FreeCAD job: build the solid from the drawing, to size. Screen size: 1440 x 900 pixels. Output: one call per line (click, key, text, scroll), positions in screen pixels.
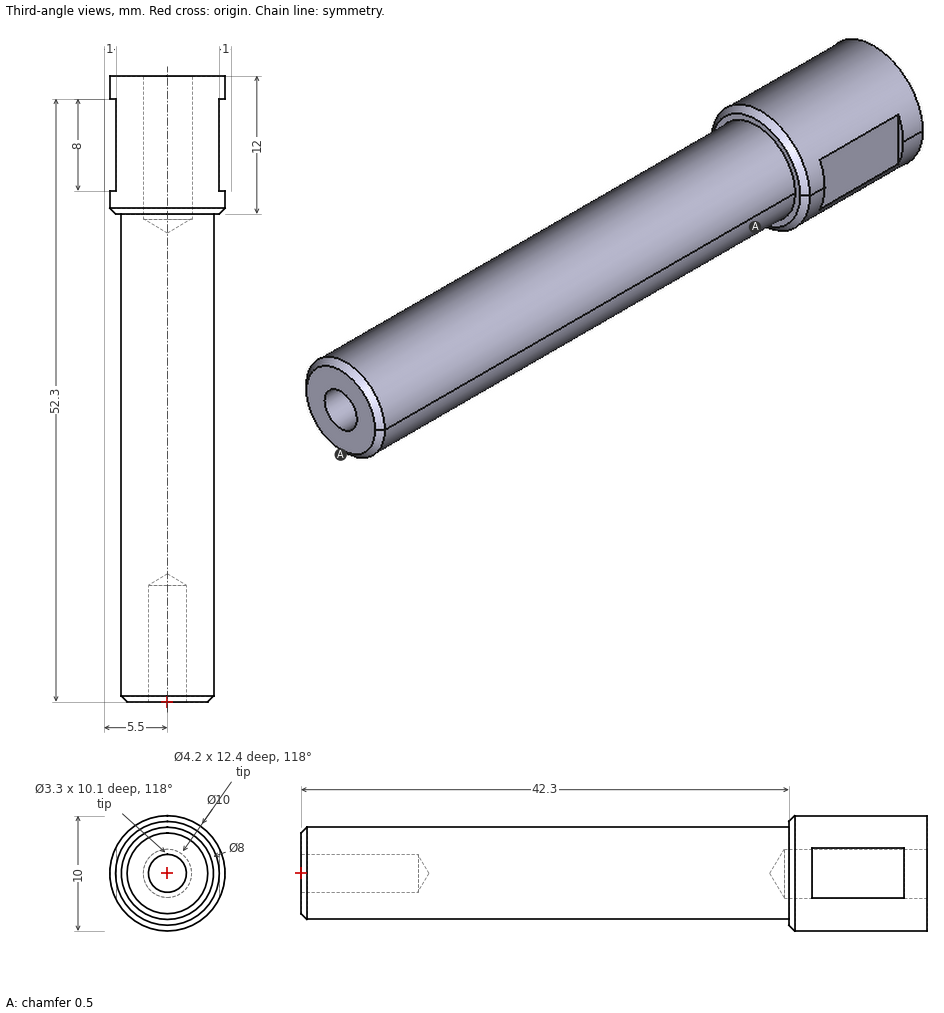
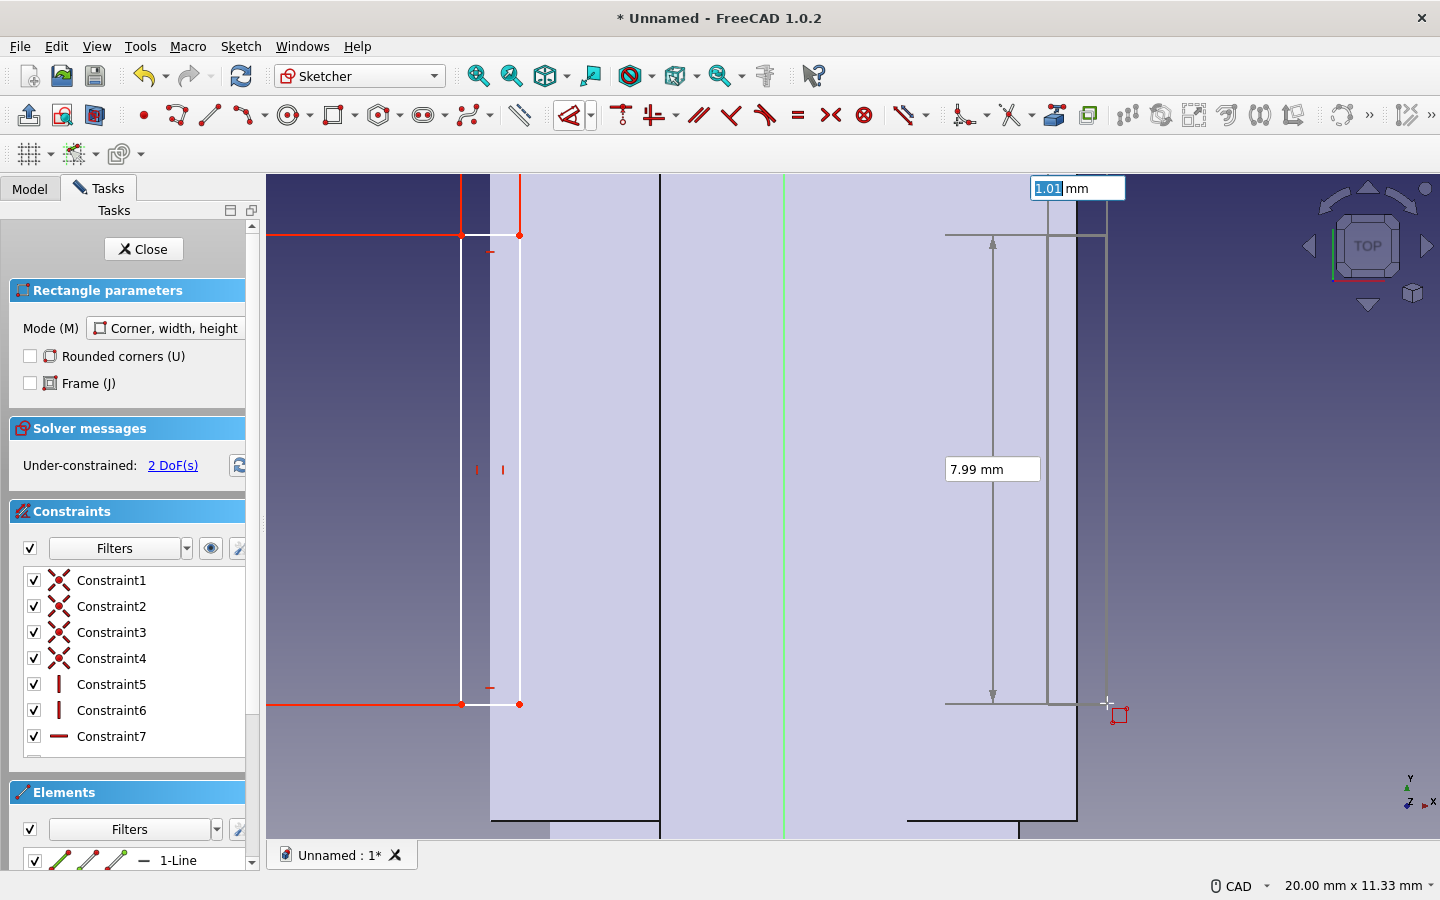
text(1)
key(Tab)
text(8)
key(Return)
key(Escape)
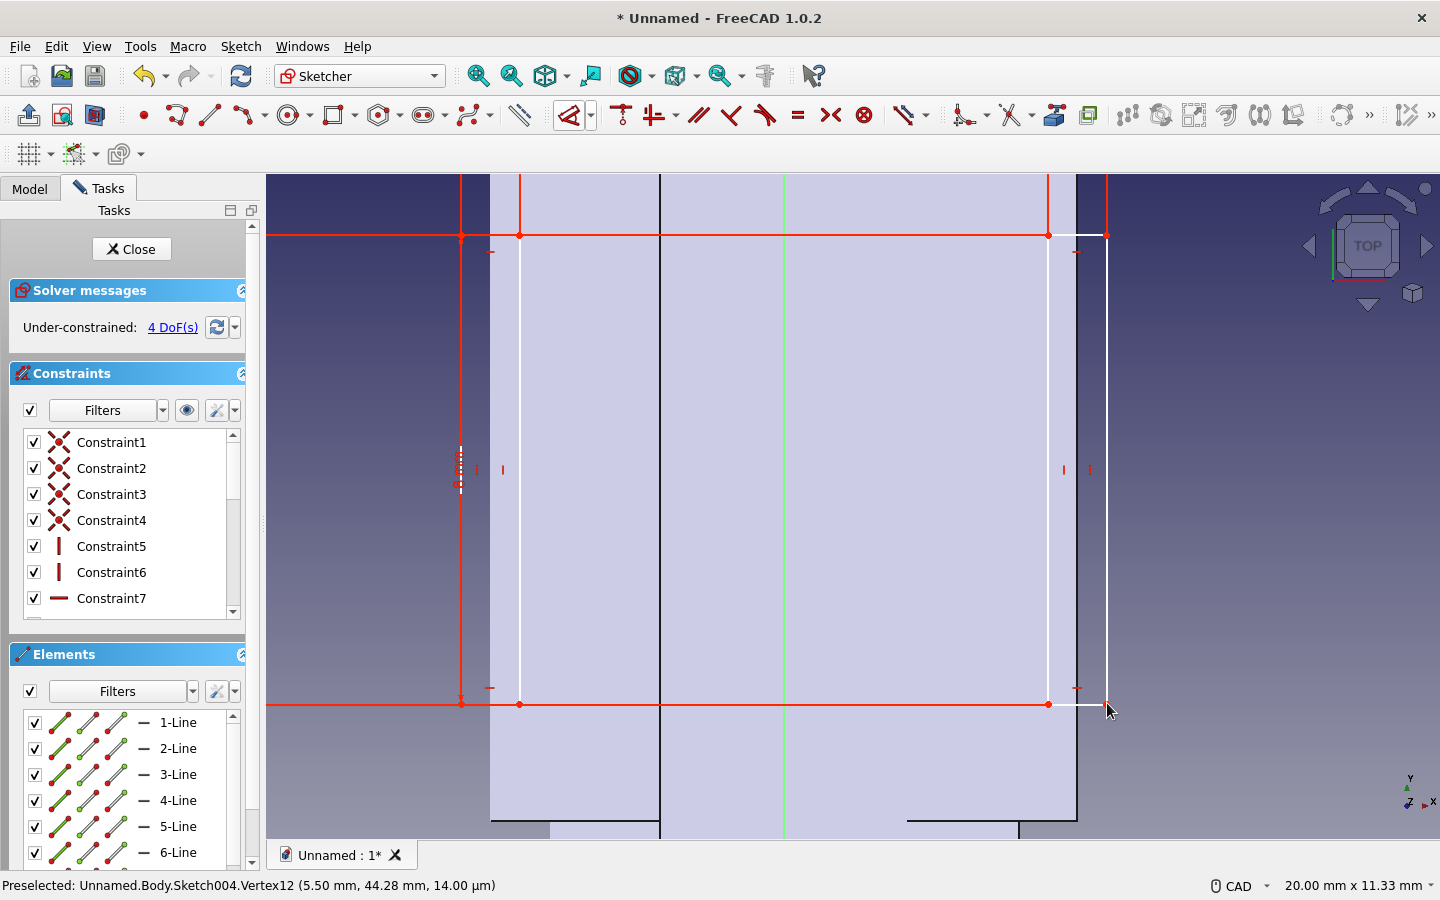
click(520, 235)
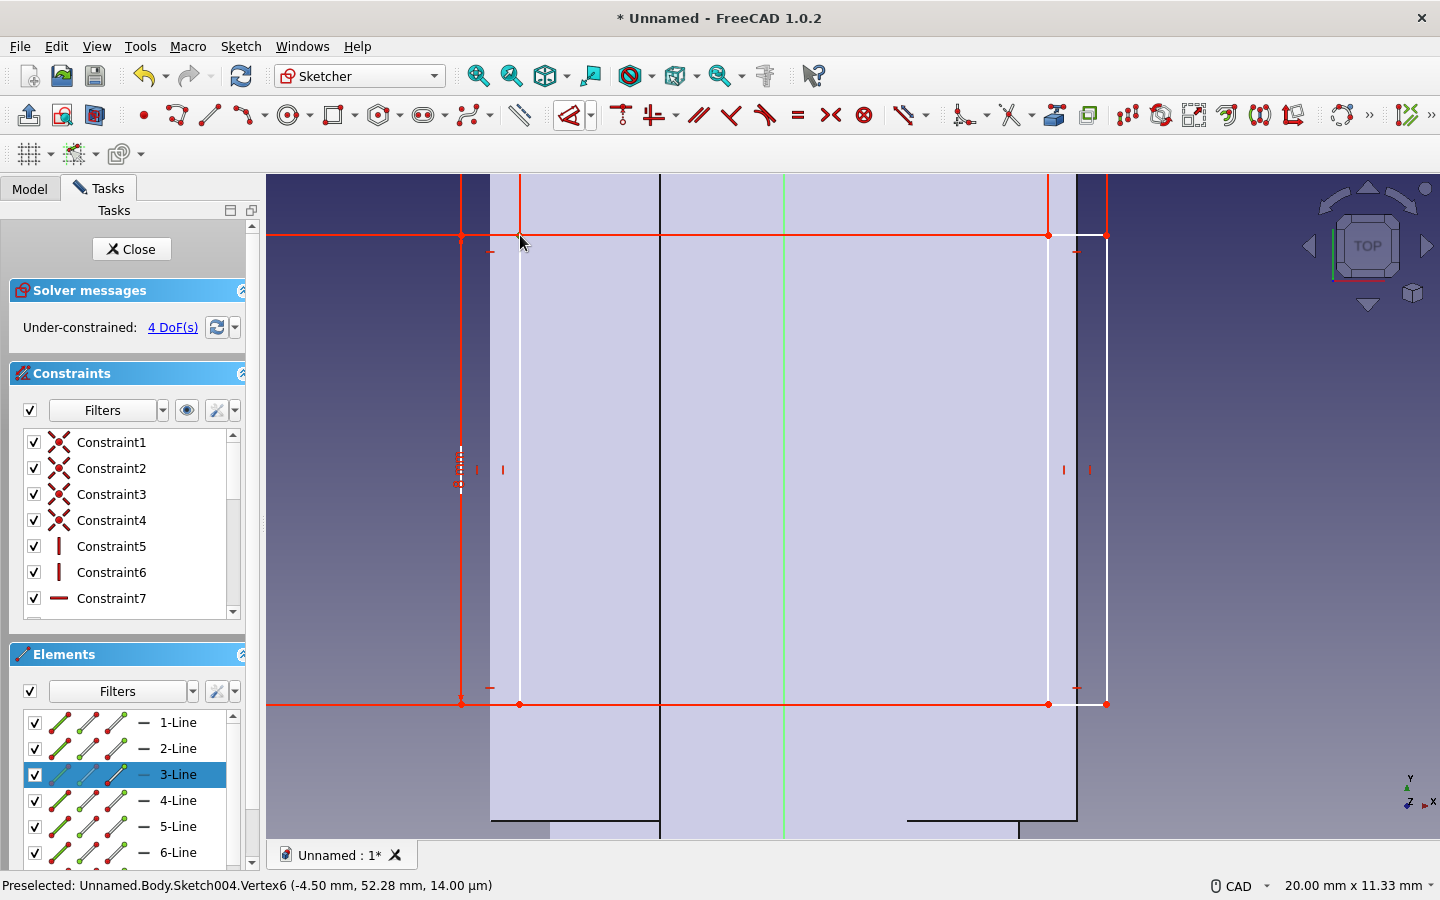
click(1048, 235)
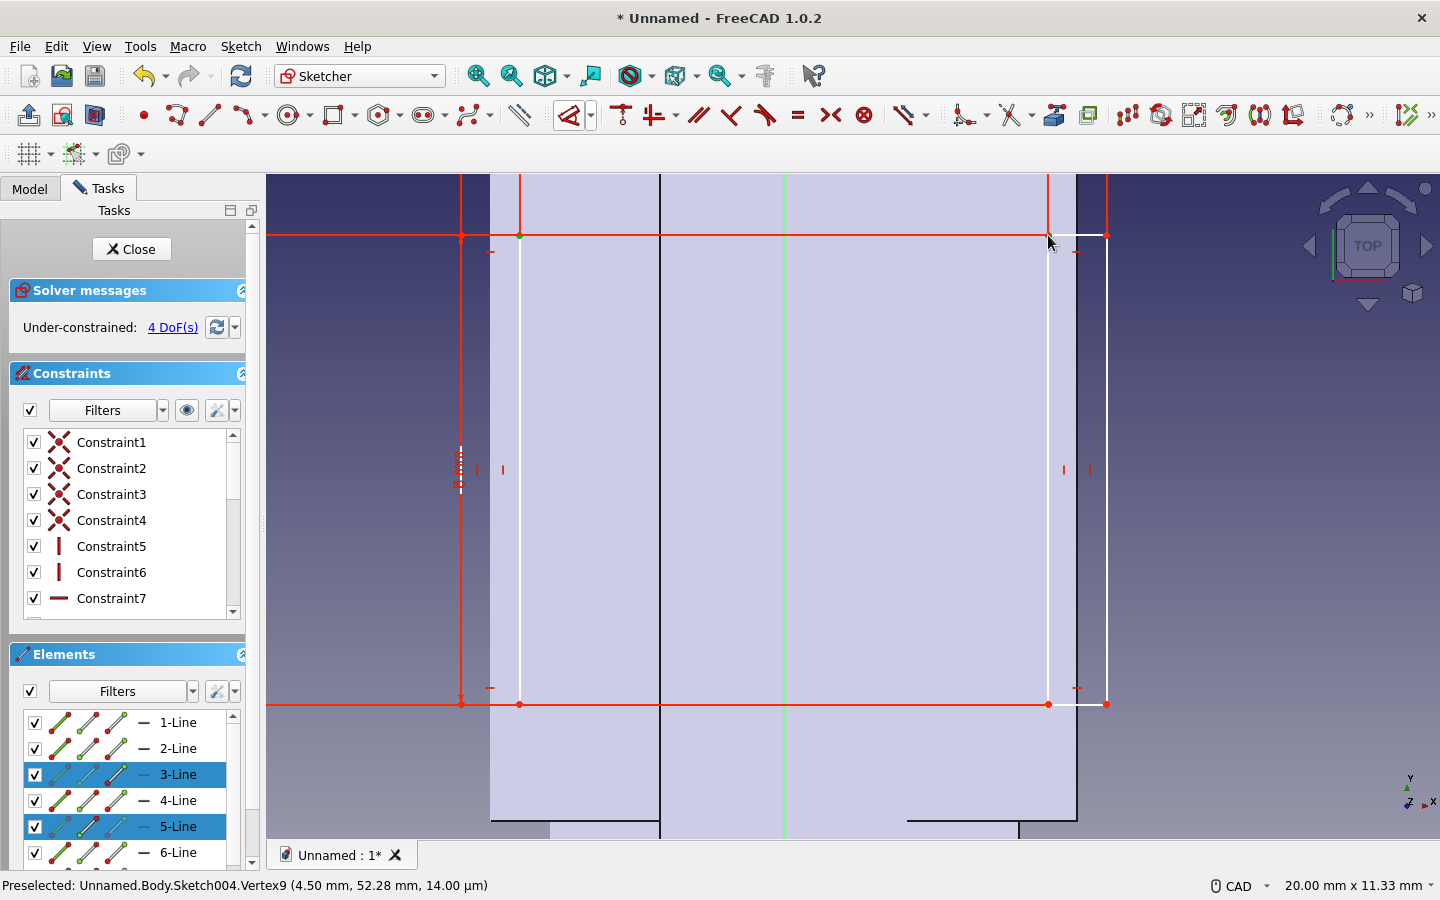
click(784, 767)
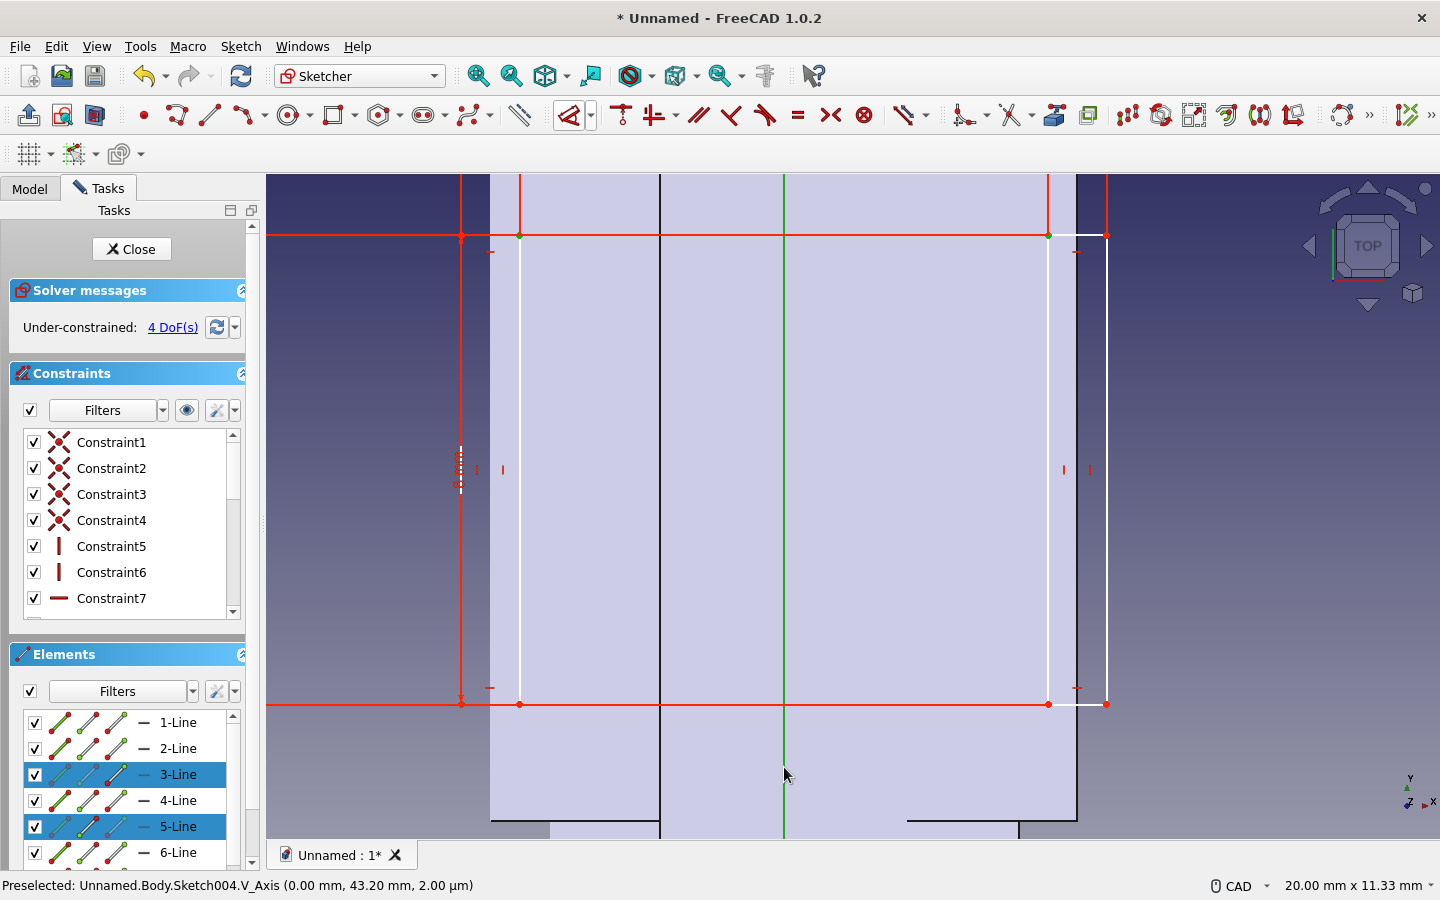
key(s)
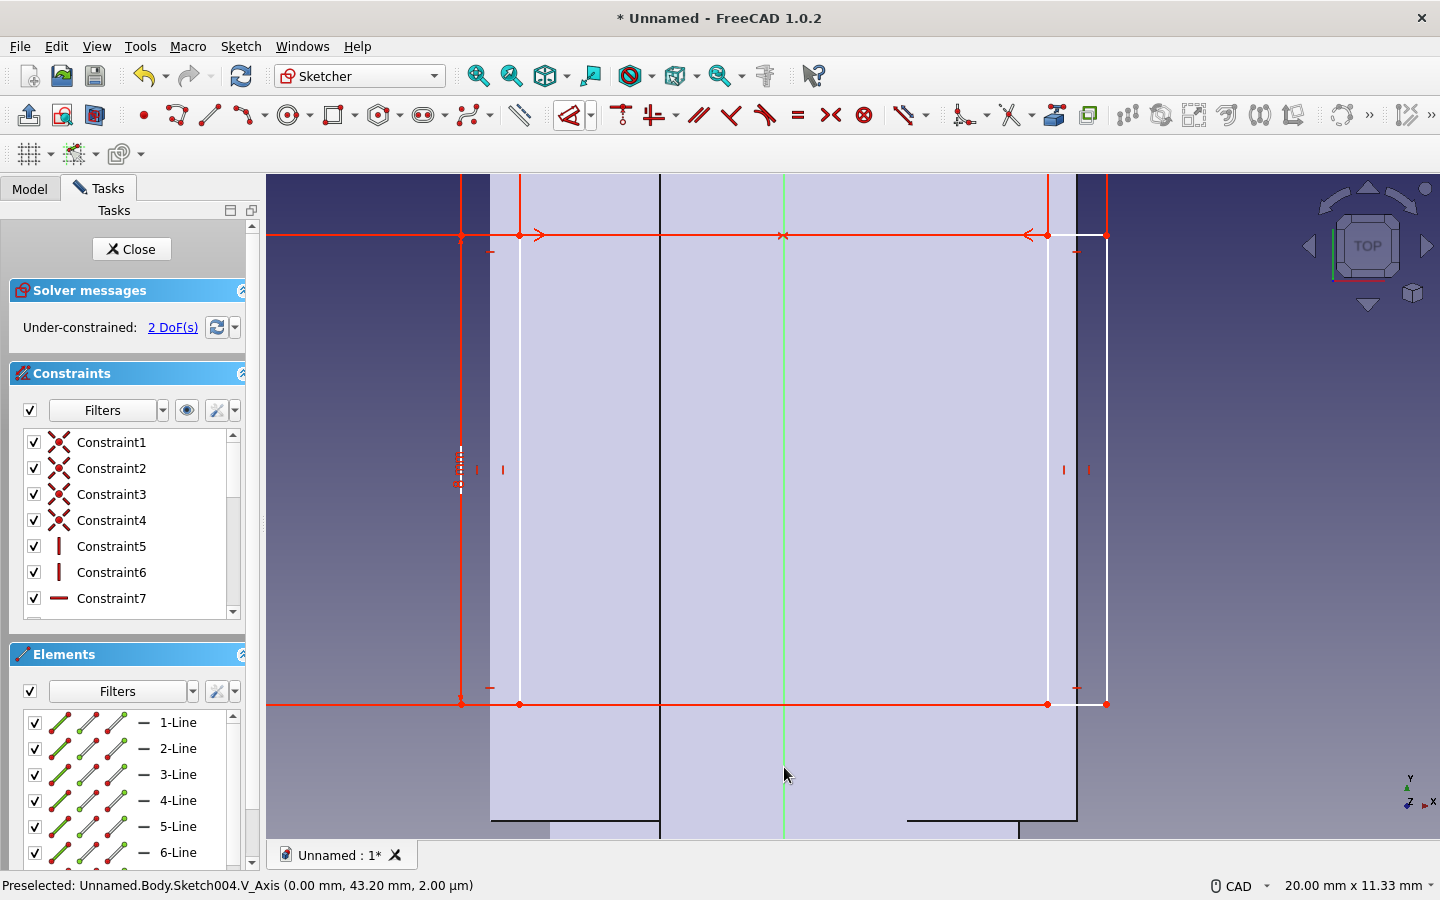
key(d)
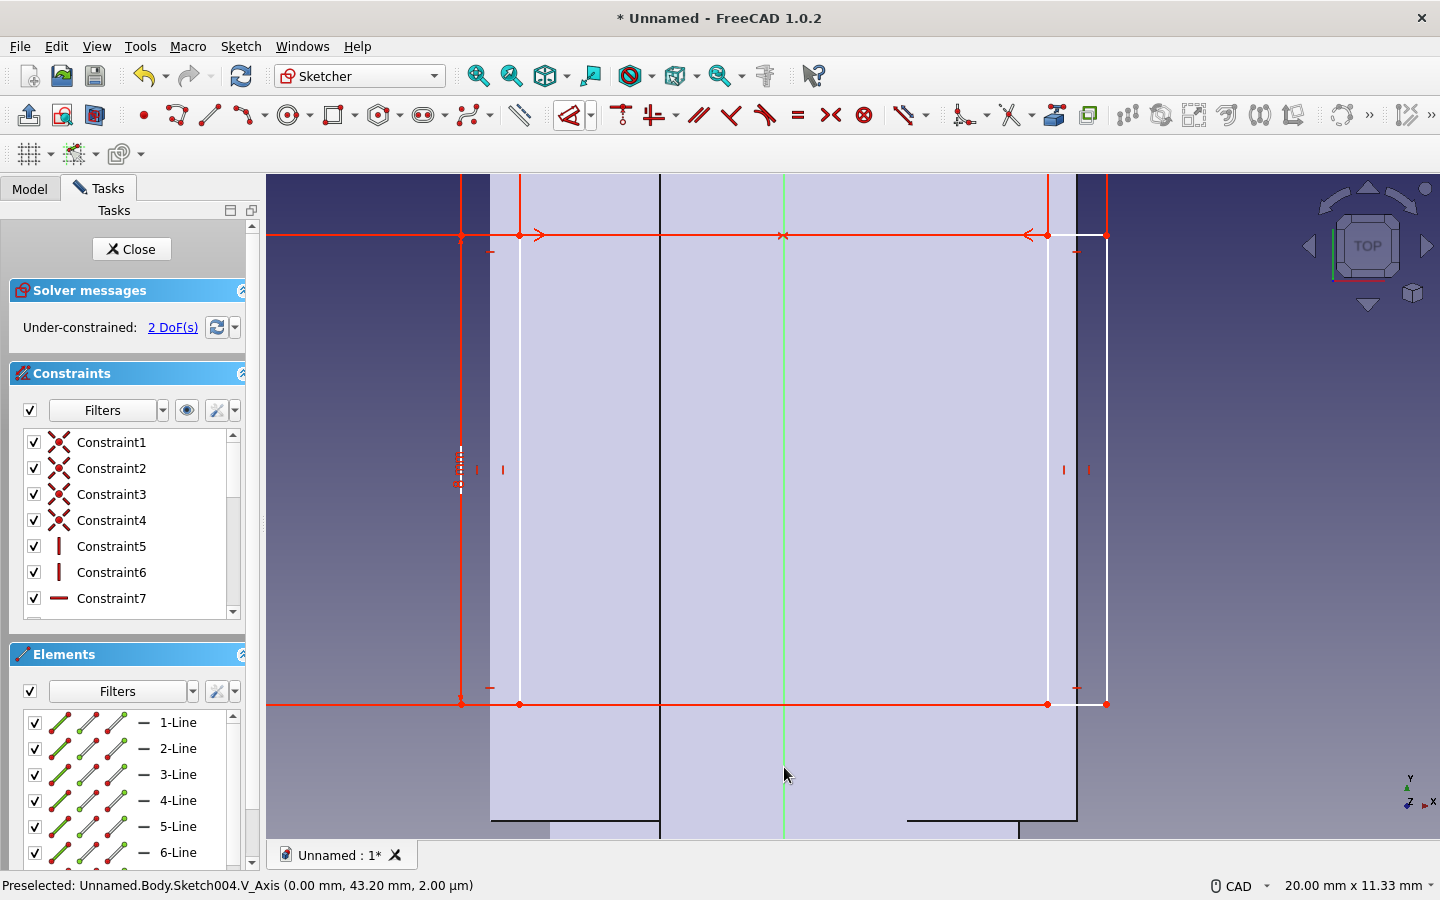
click(461, 235)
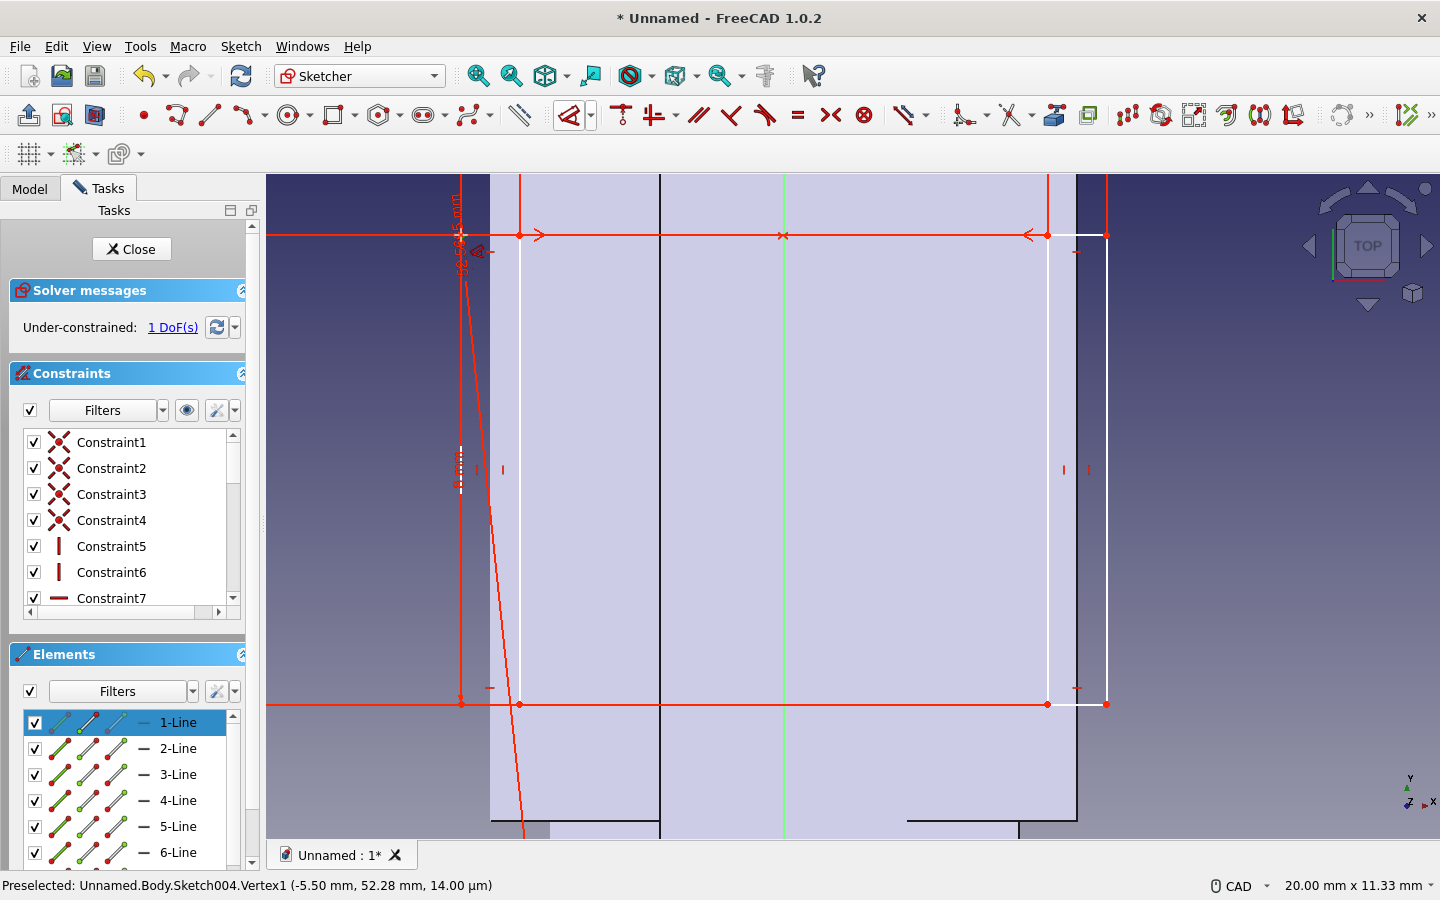
key(Escape)
key(Escape)